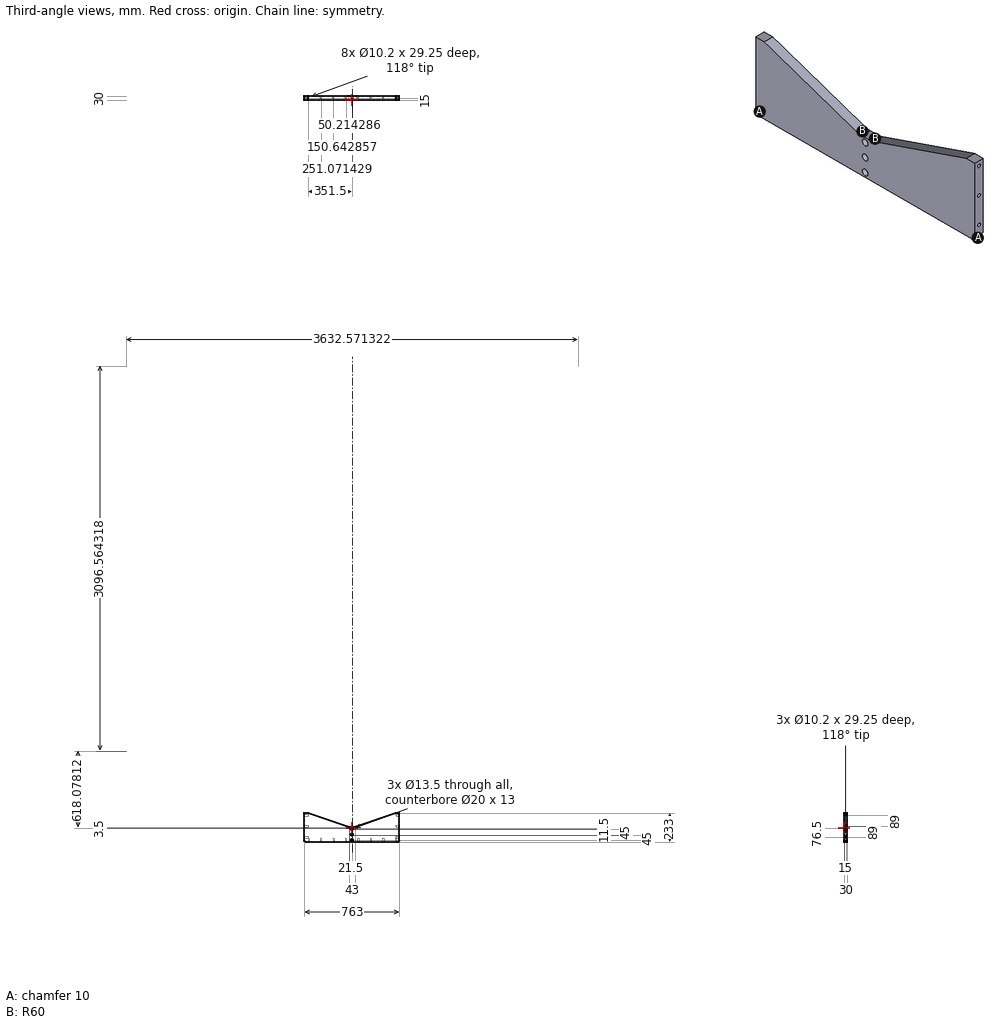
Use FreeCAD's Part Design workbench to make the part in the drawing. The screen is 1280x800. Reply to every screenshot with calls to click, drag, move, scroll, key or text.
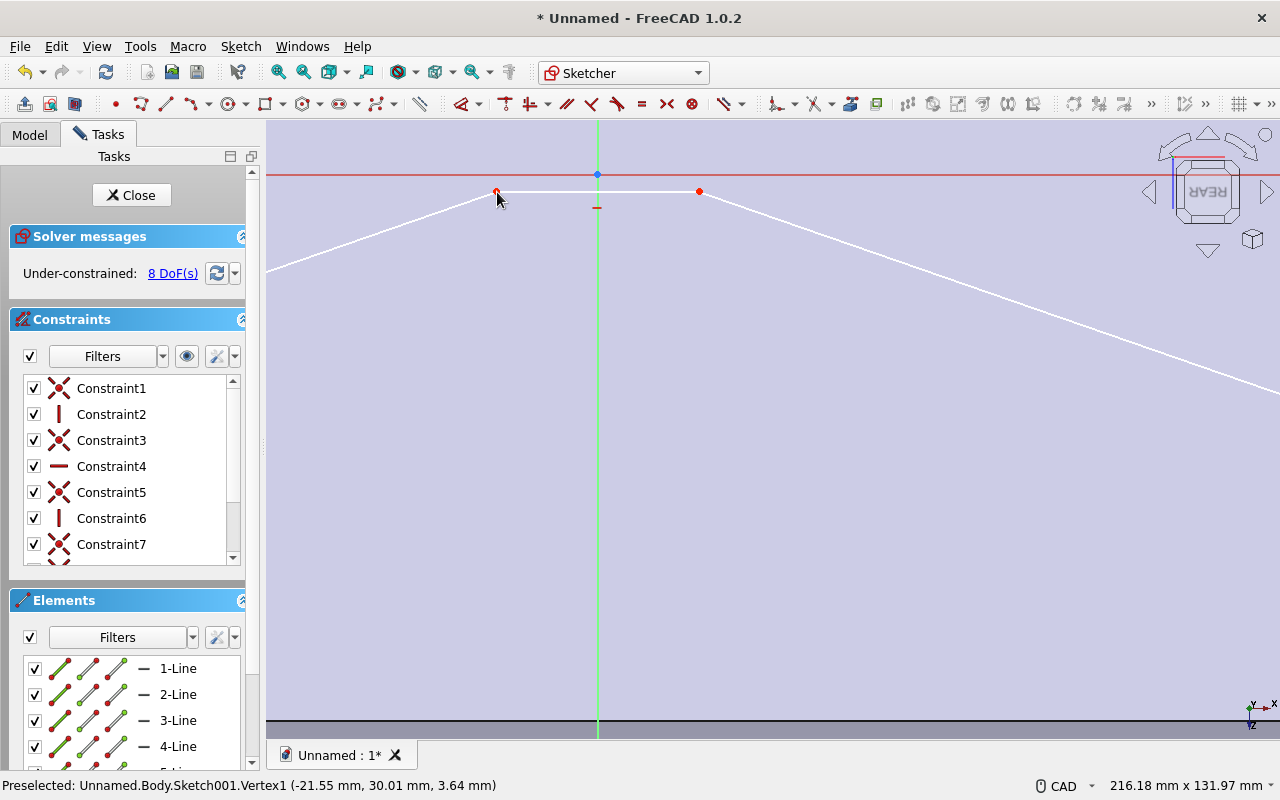
scroll(707, 192, down, 18)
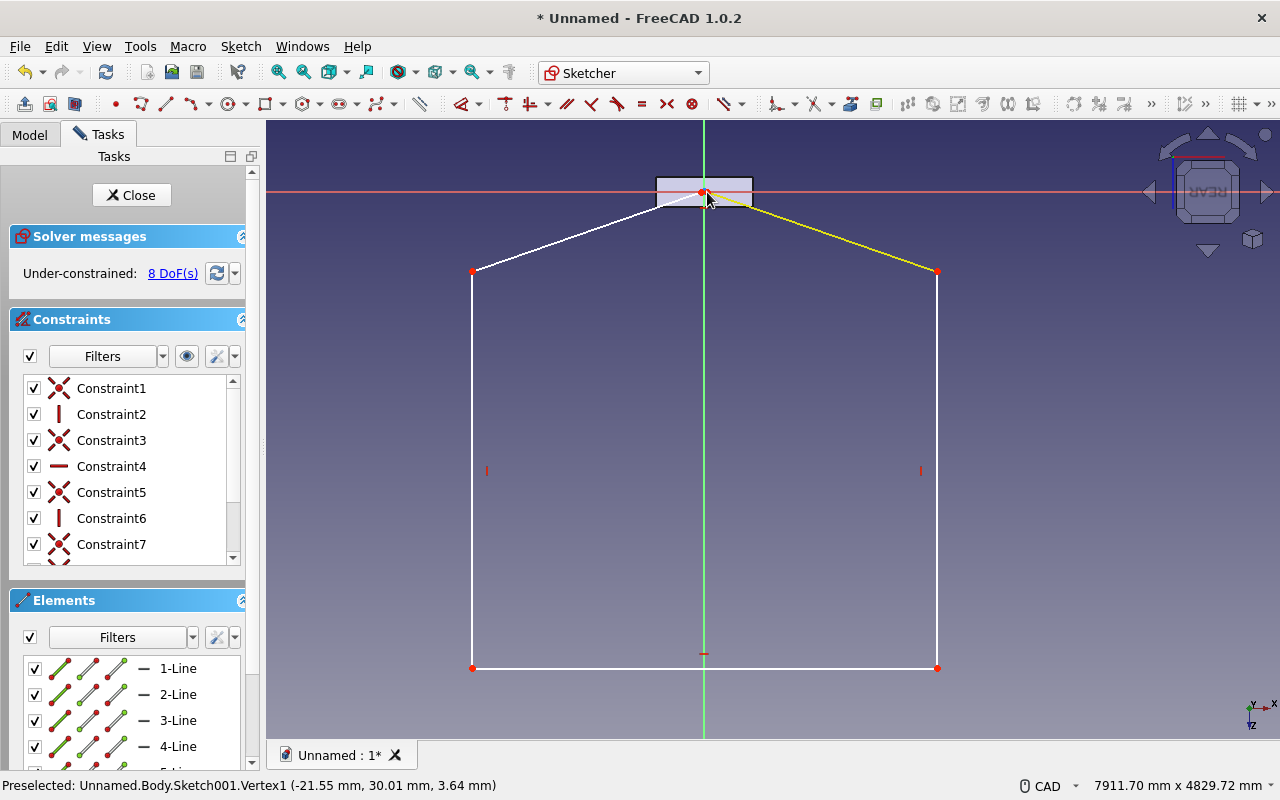
click(472, 272)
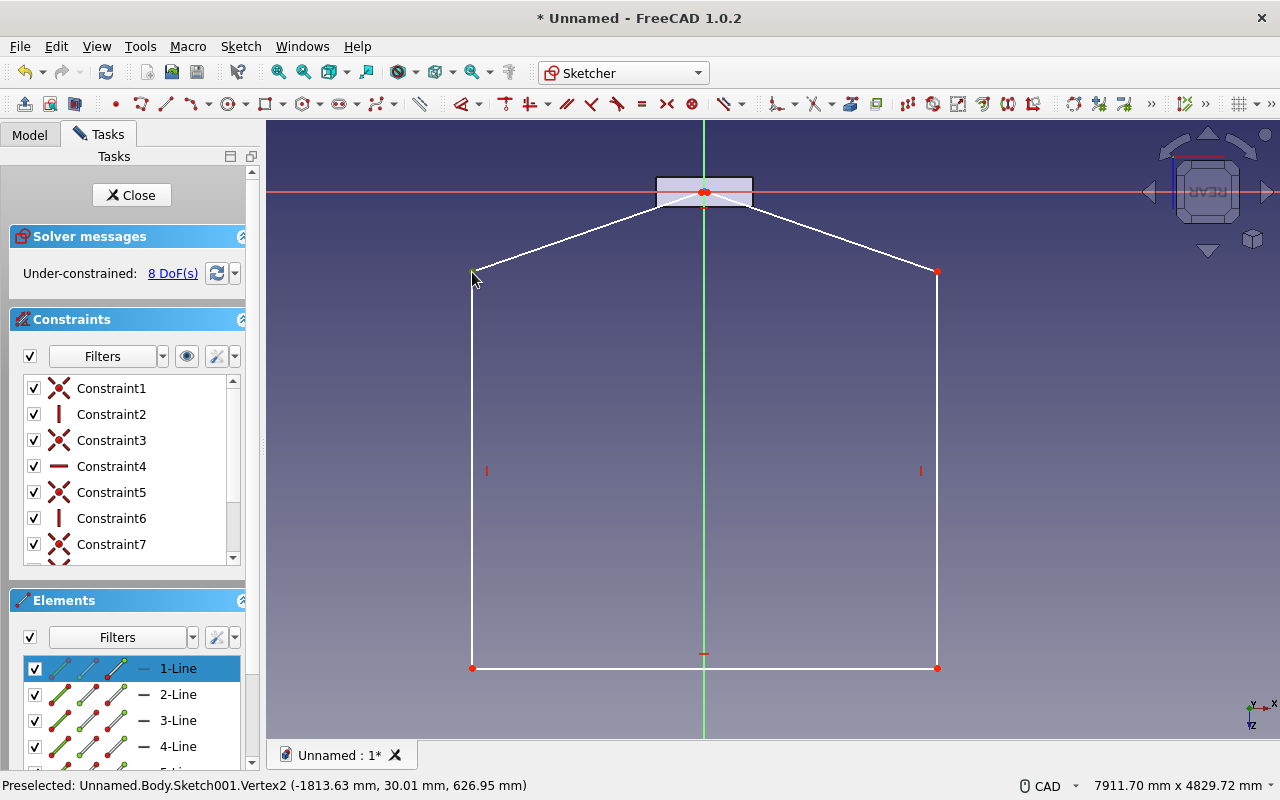
click(937, 272)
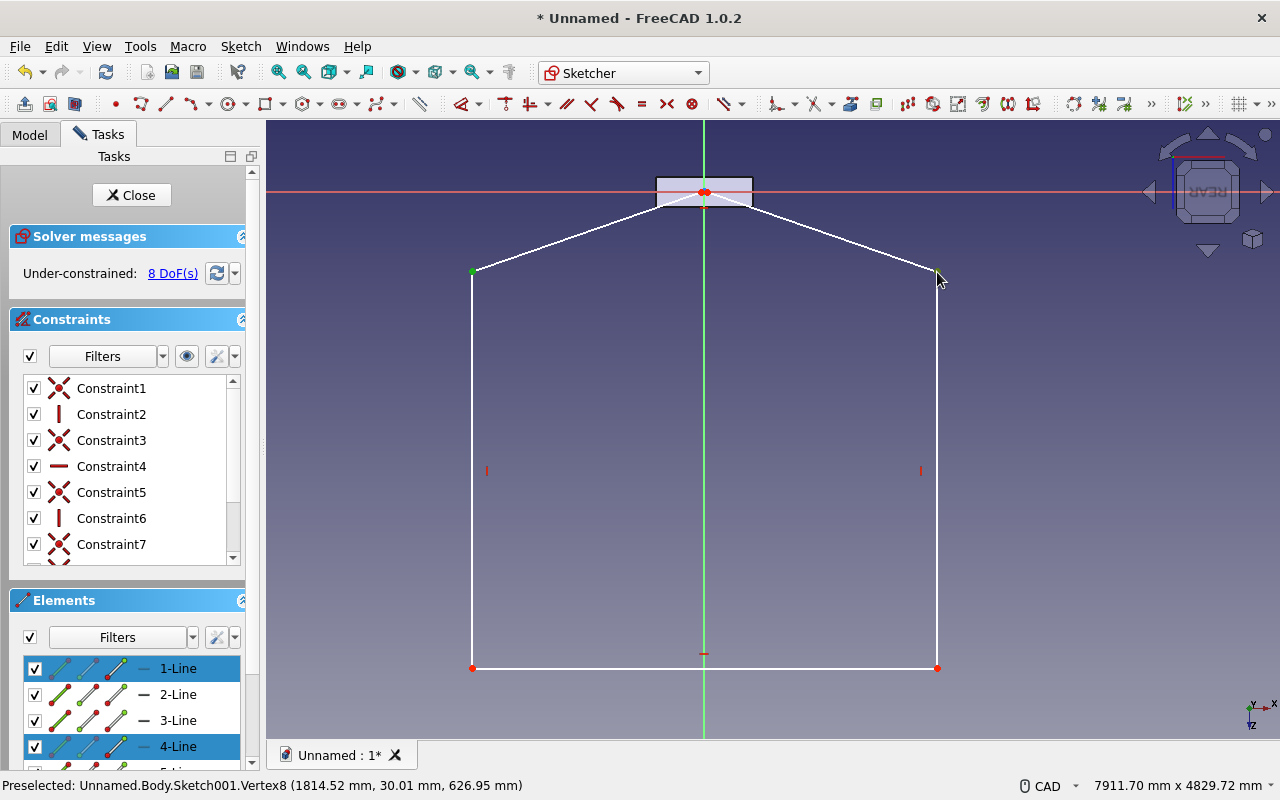
click(704, 631)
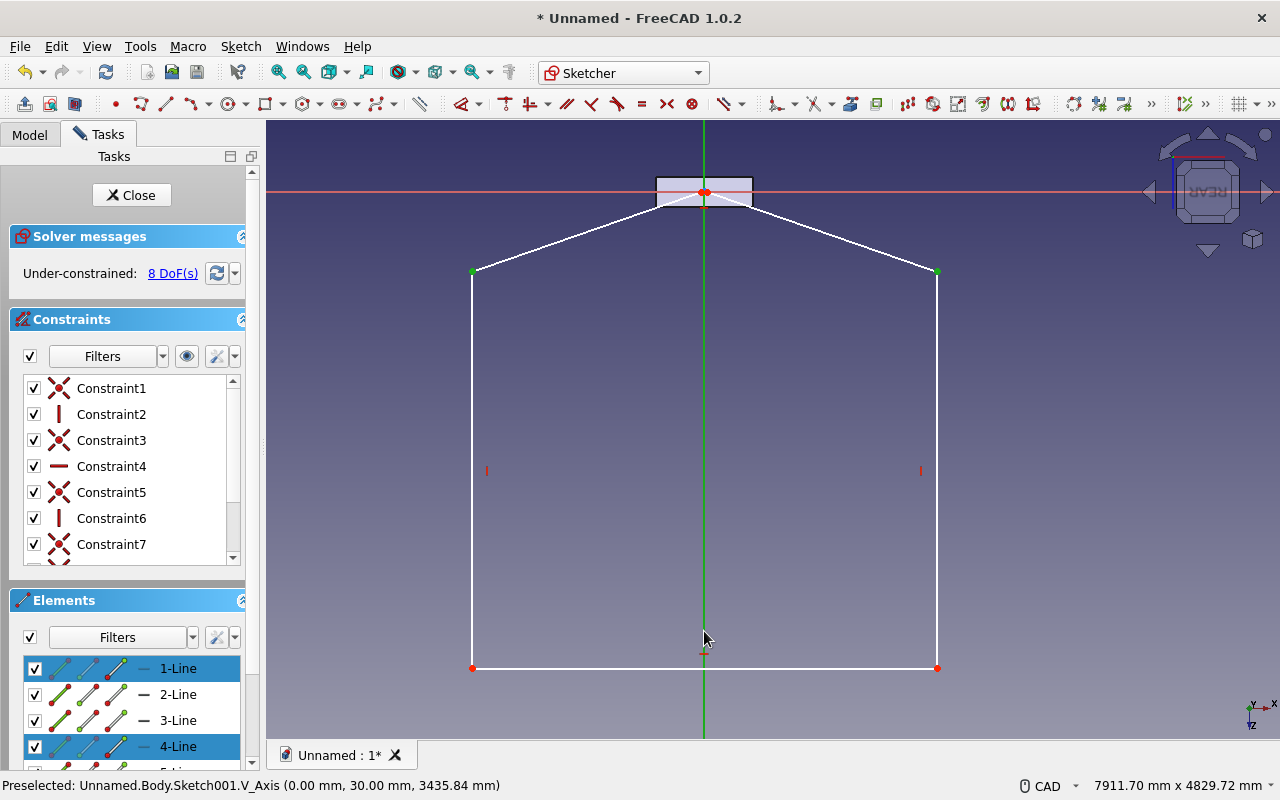
key(s)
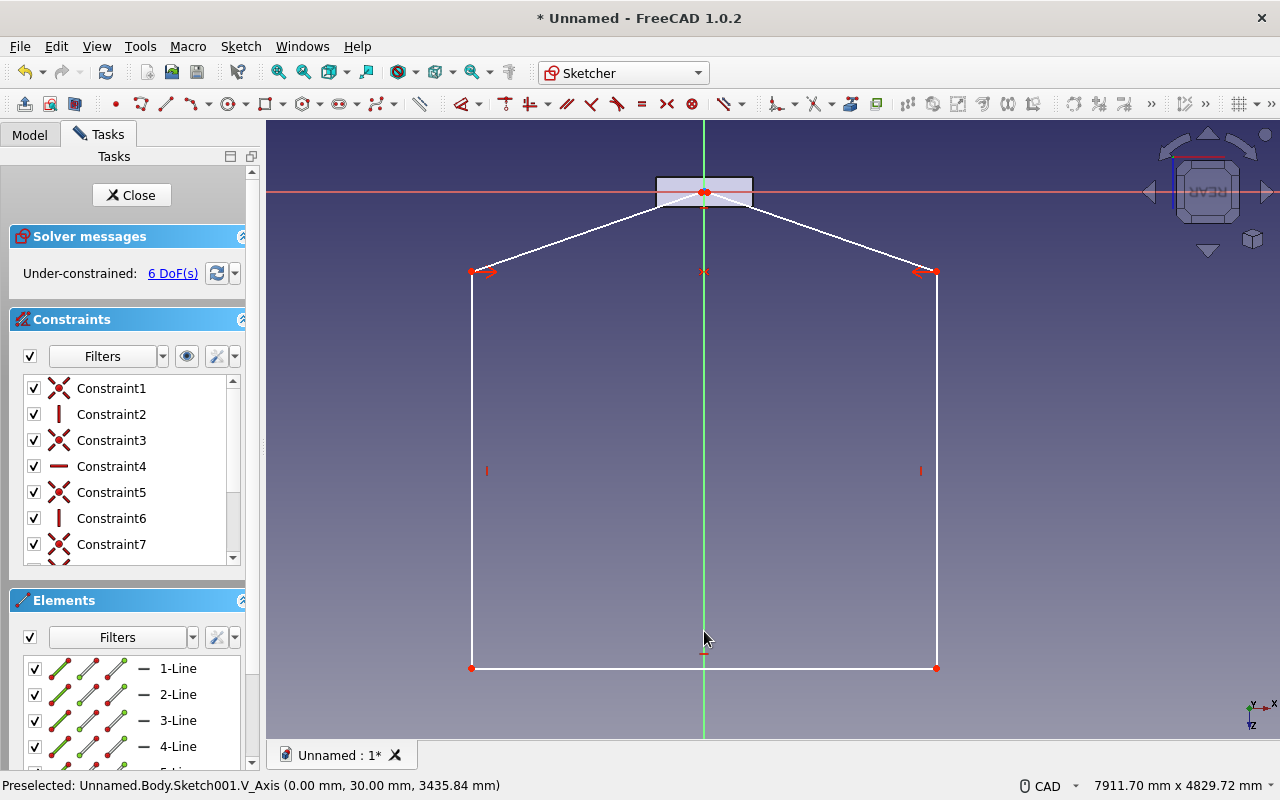
key(d)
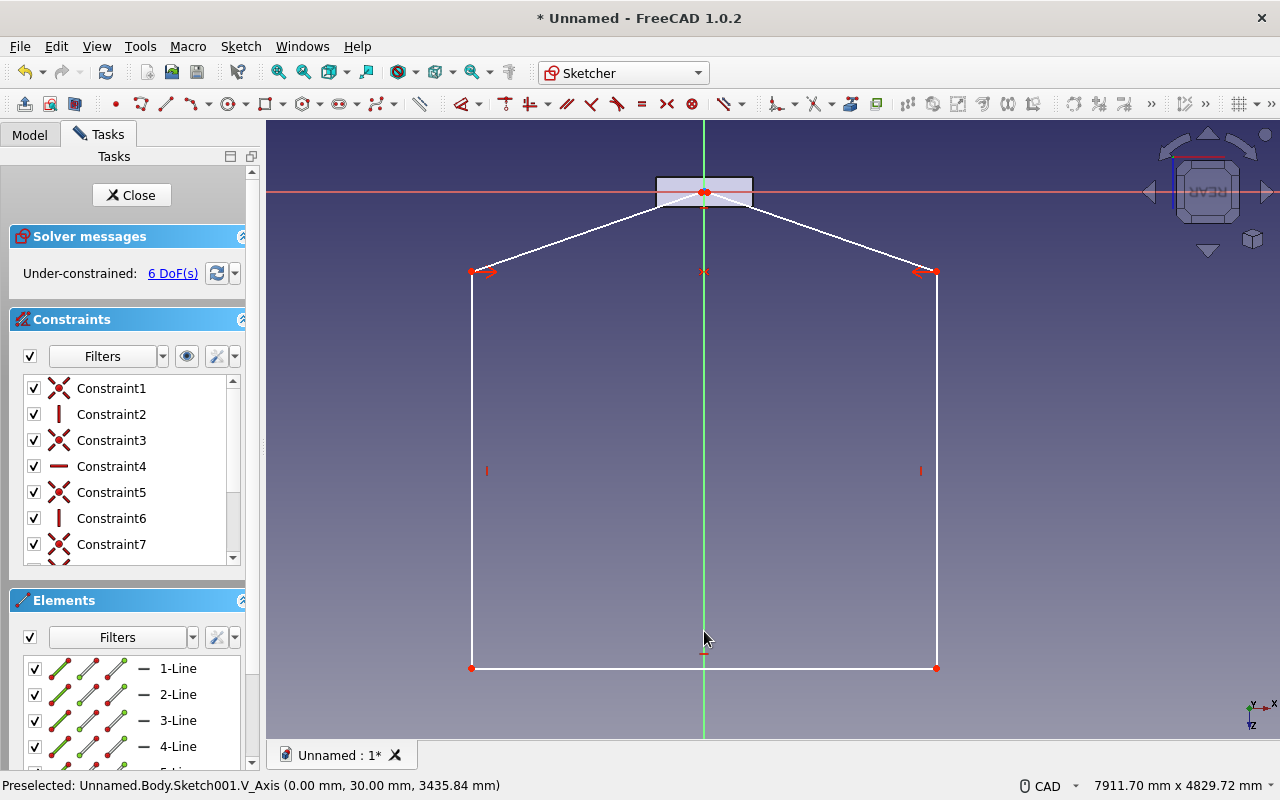
scroll(704, 192, up, 10)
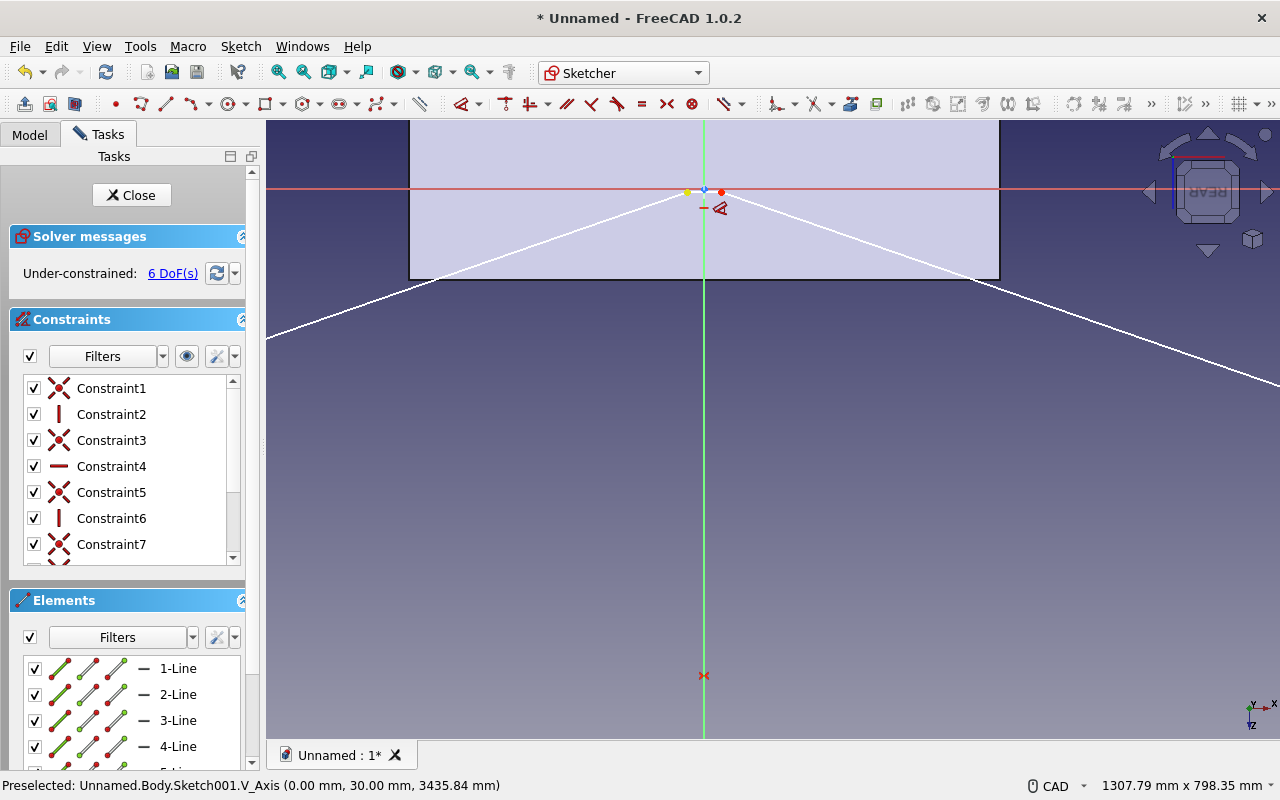
click(700, 192)
click(690, 158)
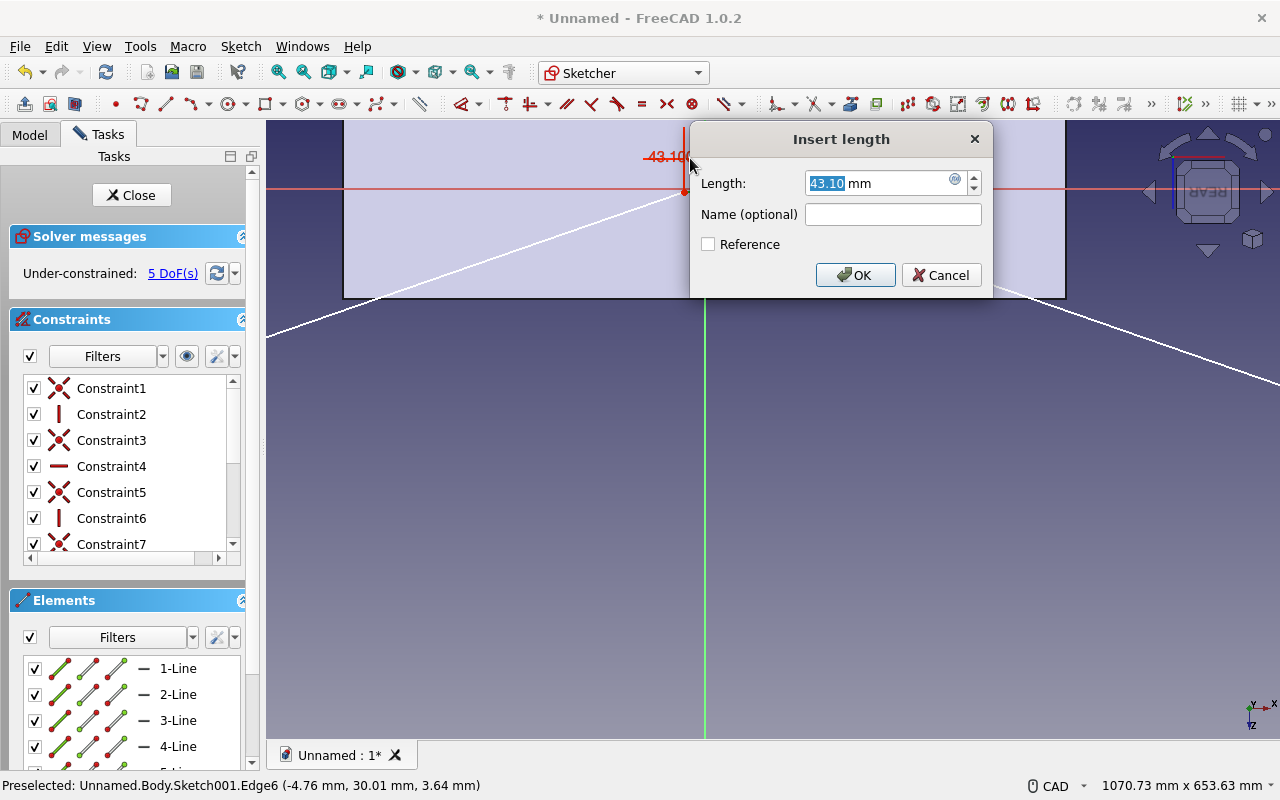
text(43)
key(Return)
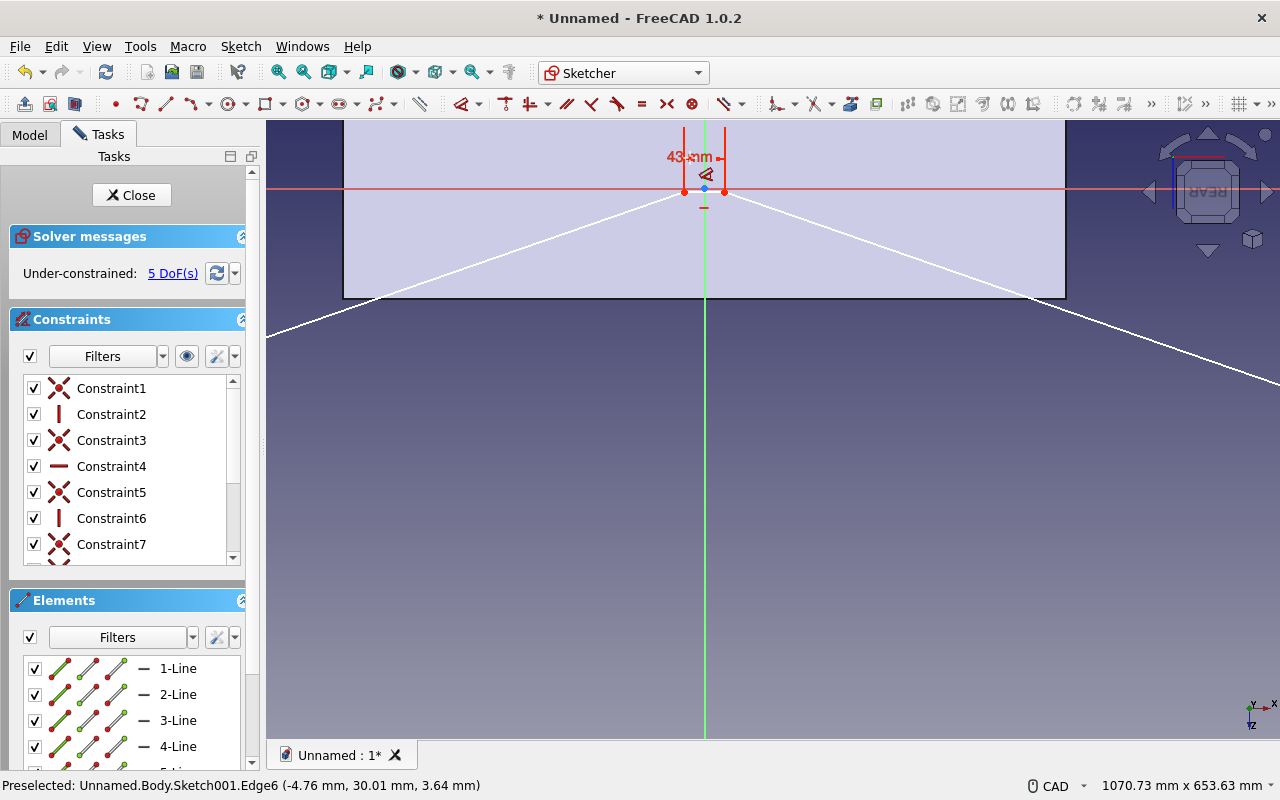
scroll(684, 192, up, 13)